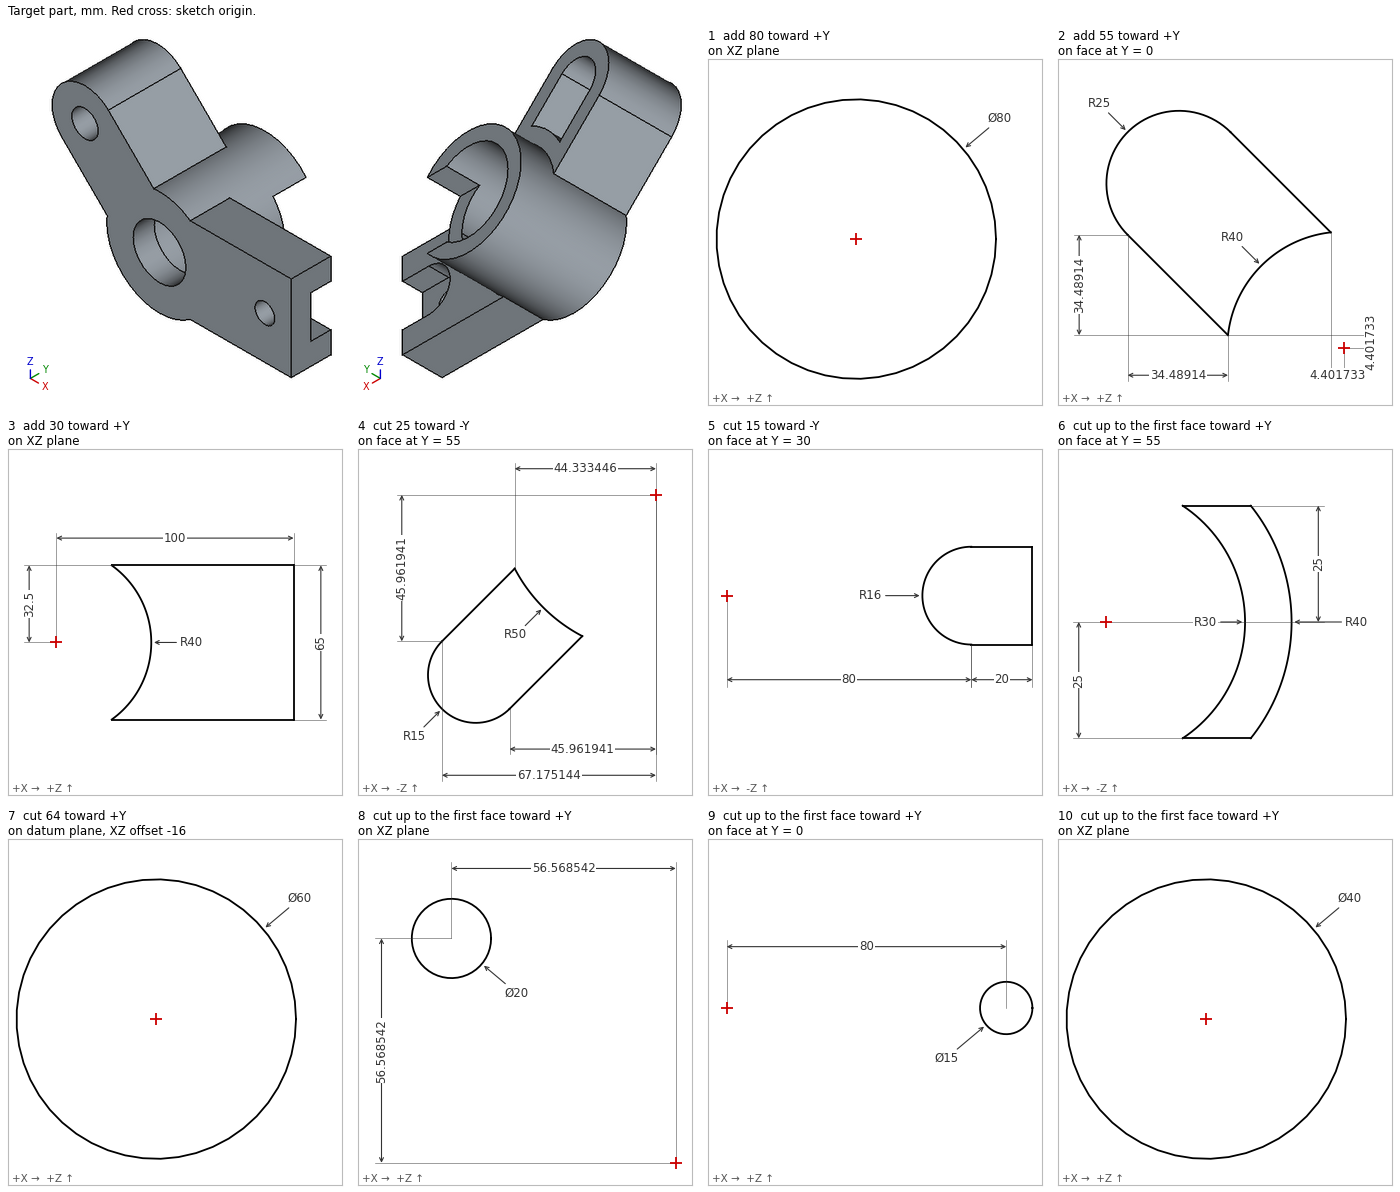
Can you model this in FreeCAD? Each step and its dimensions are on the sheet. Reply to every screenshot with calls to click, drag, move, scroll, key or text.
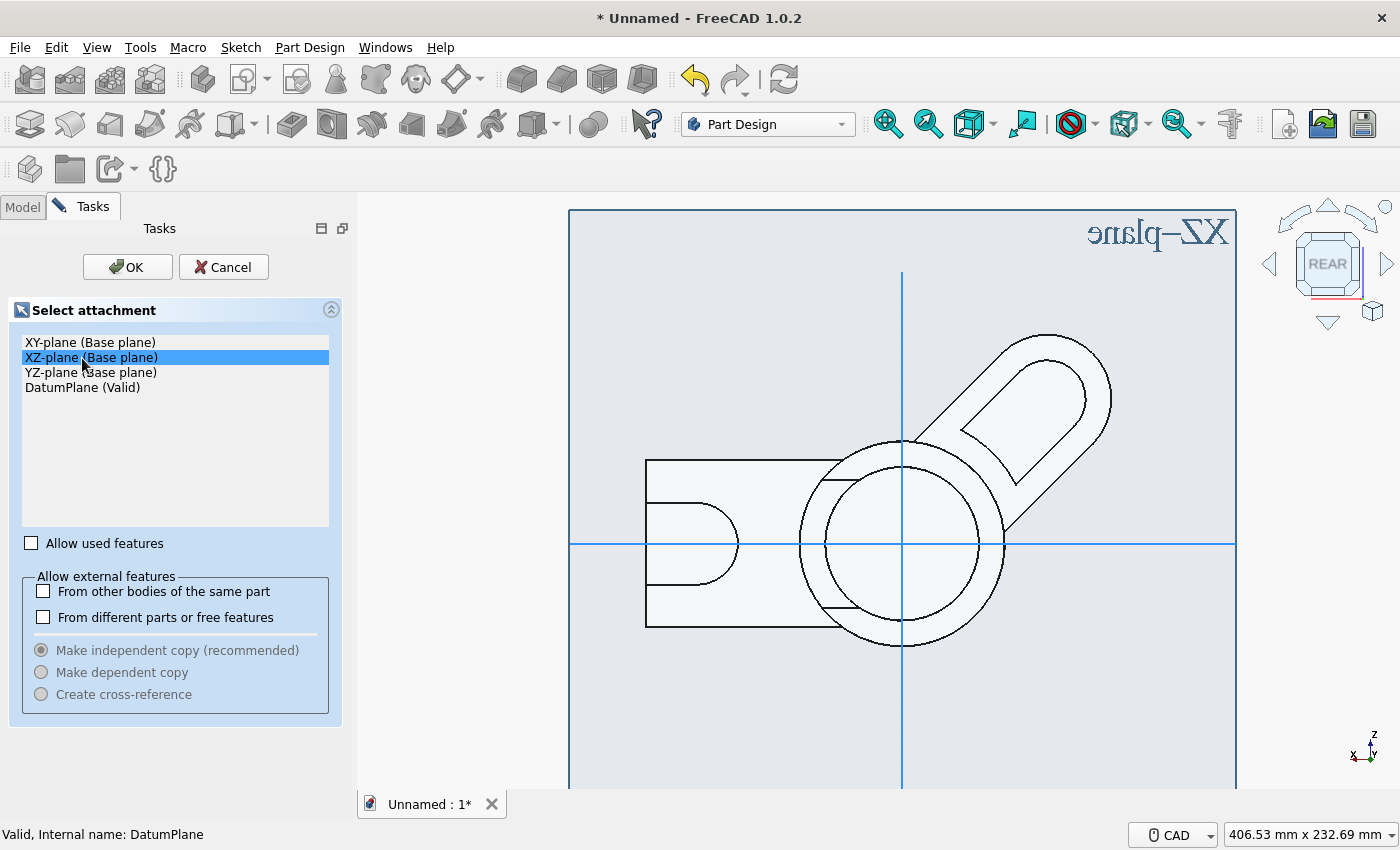
click(128, 267)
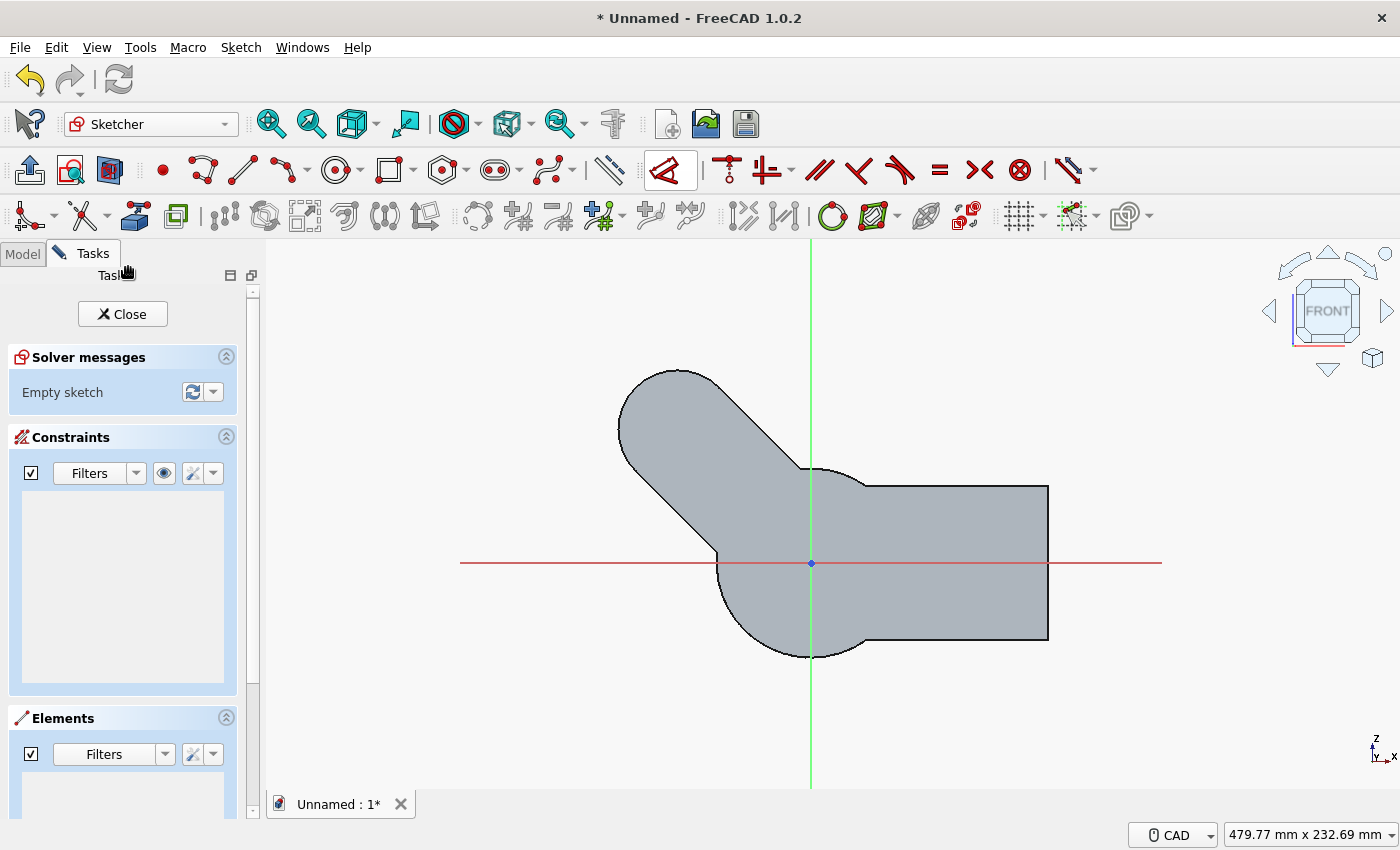
scroll(664, 416, up, 10)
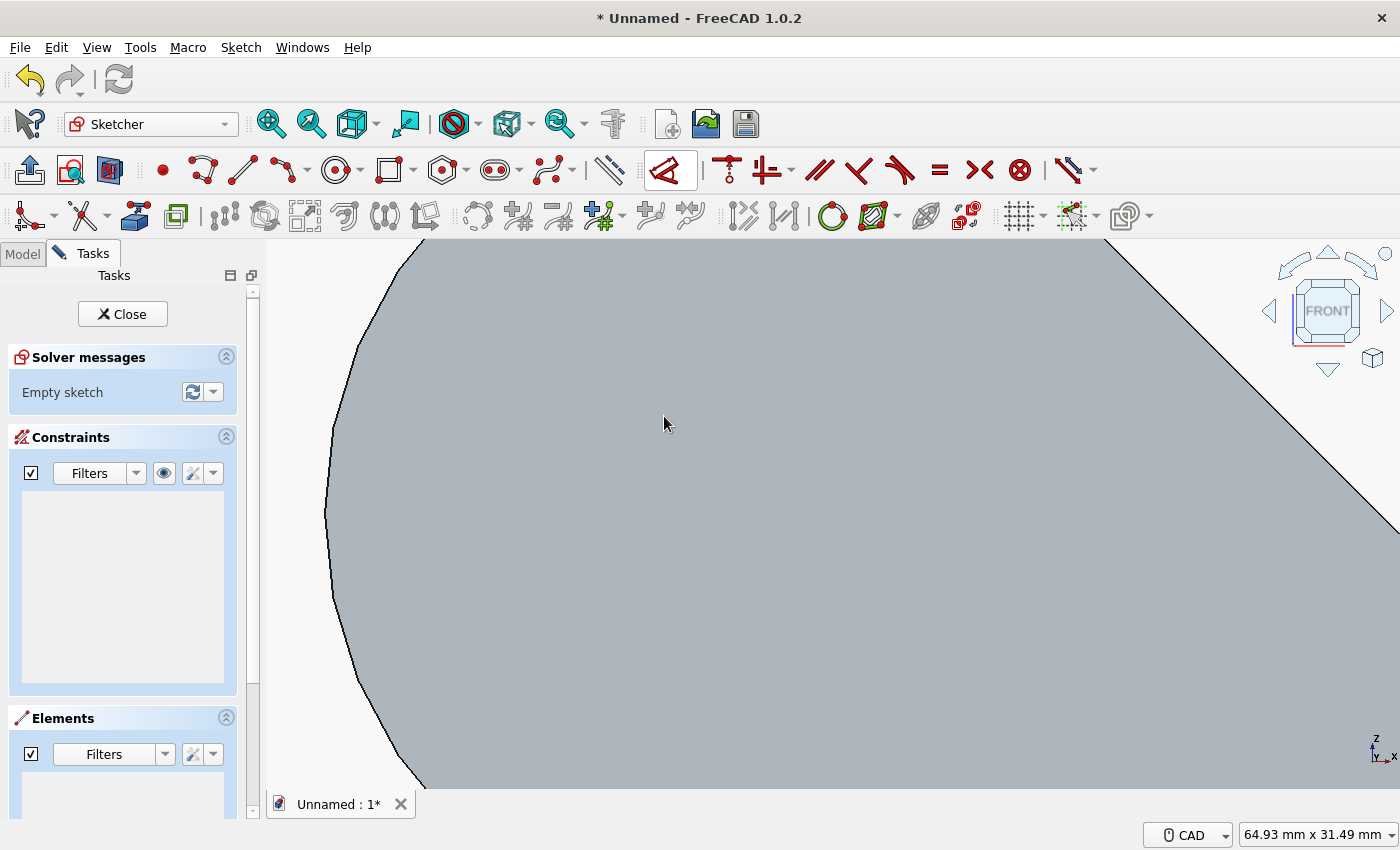
click(336, 170)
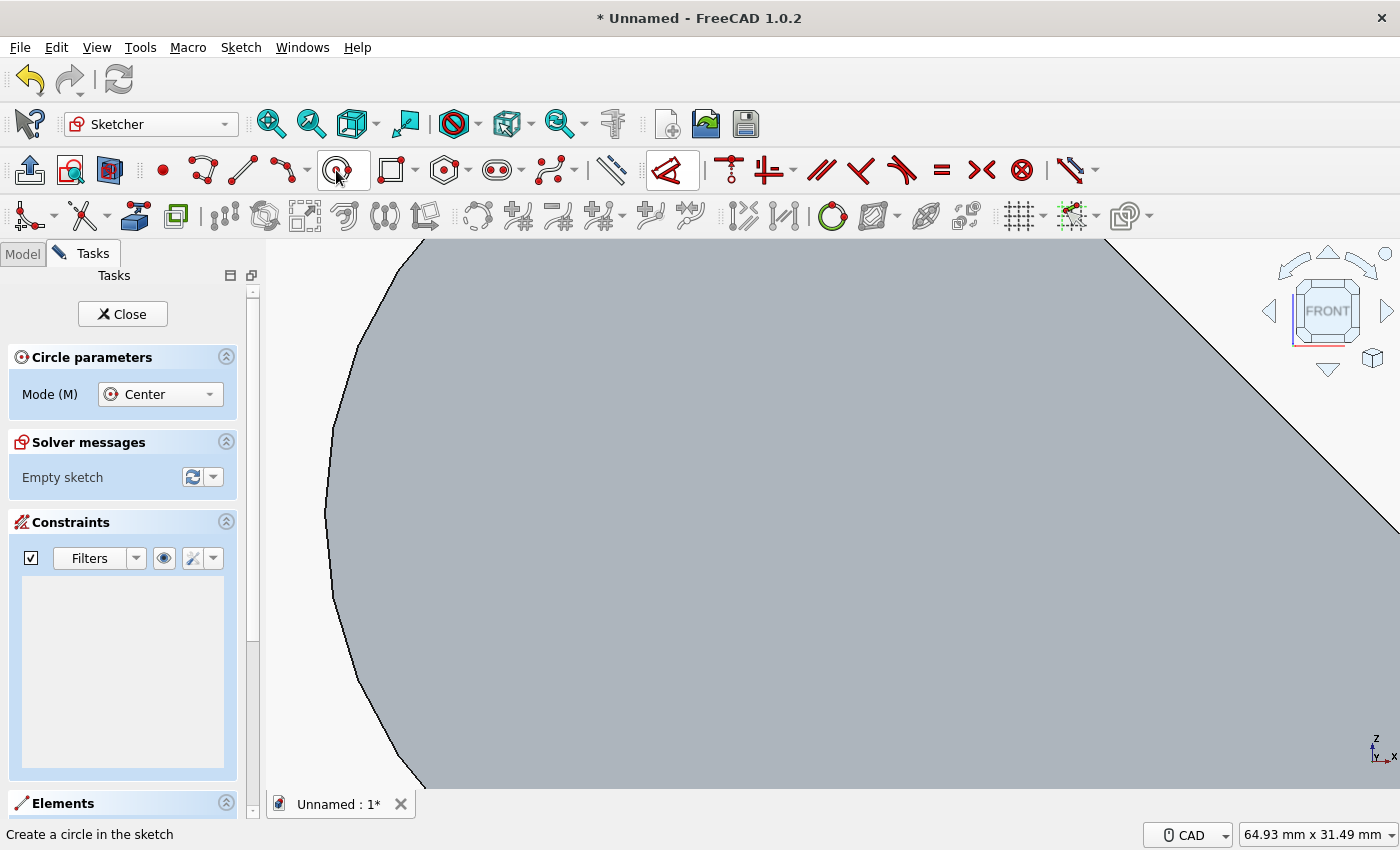
click(762, 513)
click(885, 390)
key(Escape)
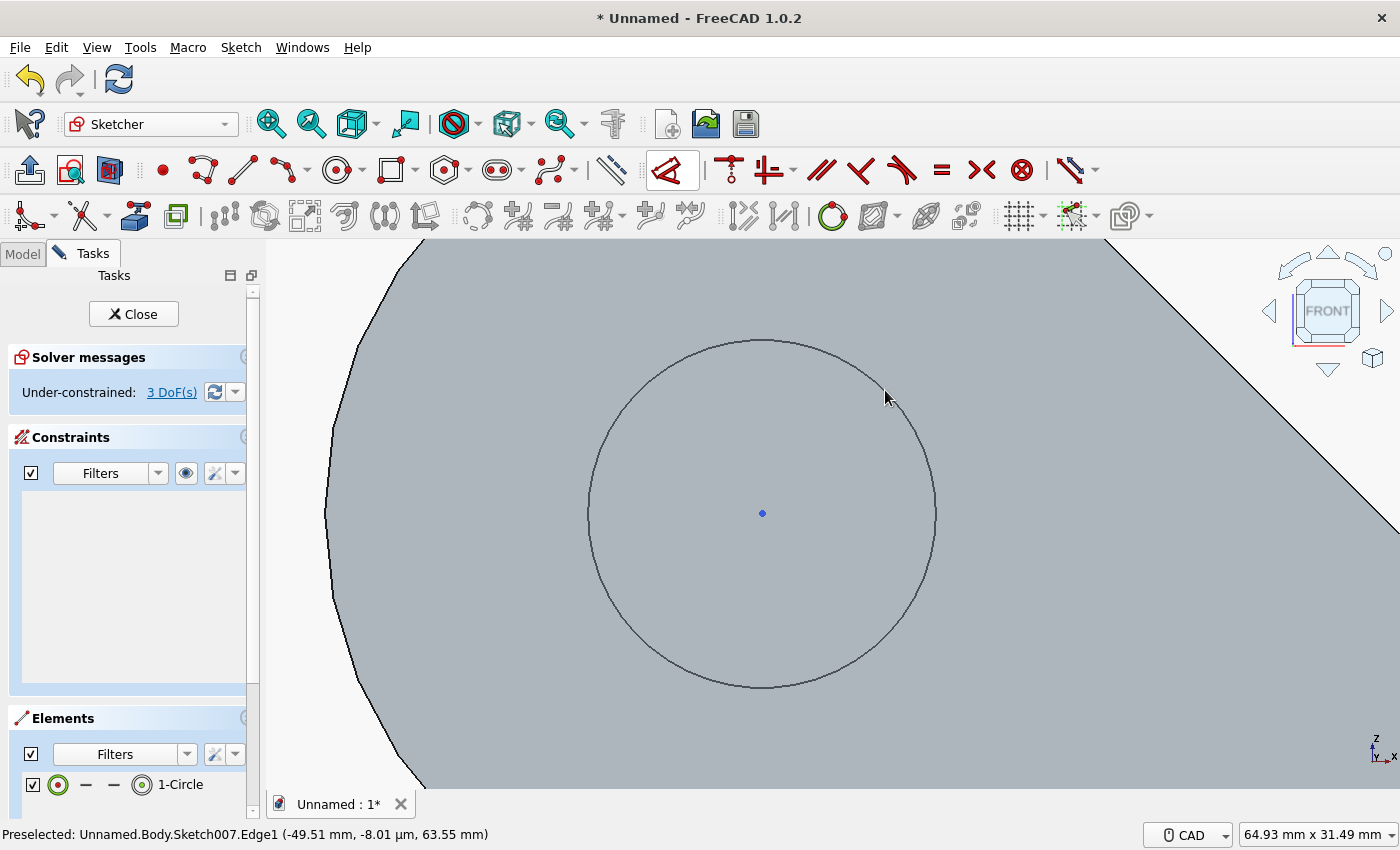
click(885, 391)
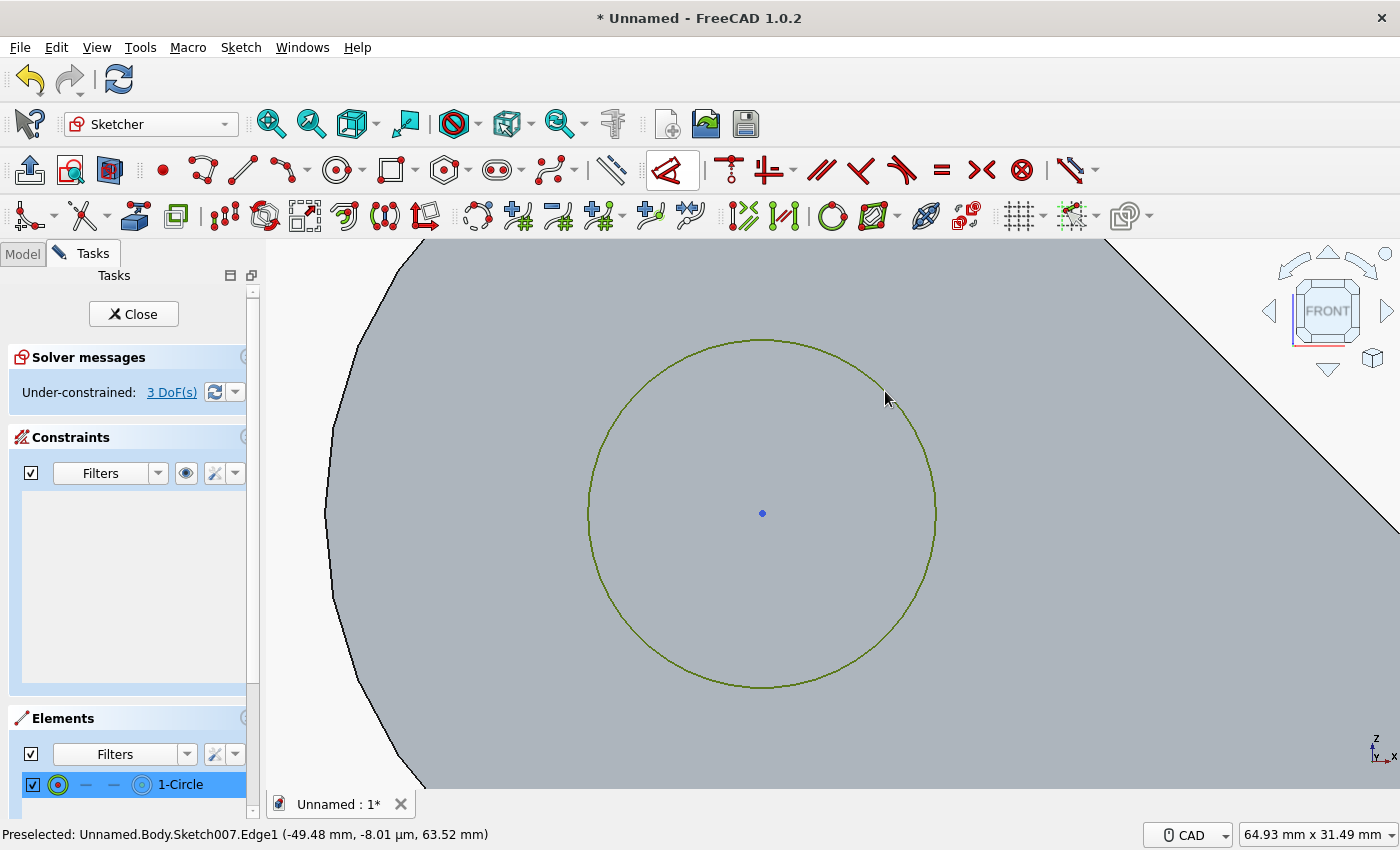
click(694, 170)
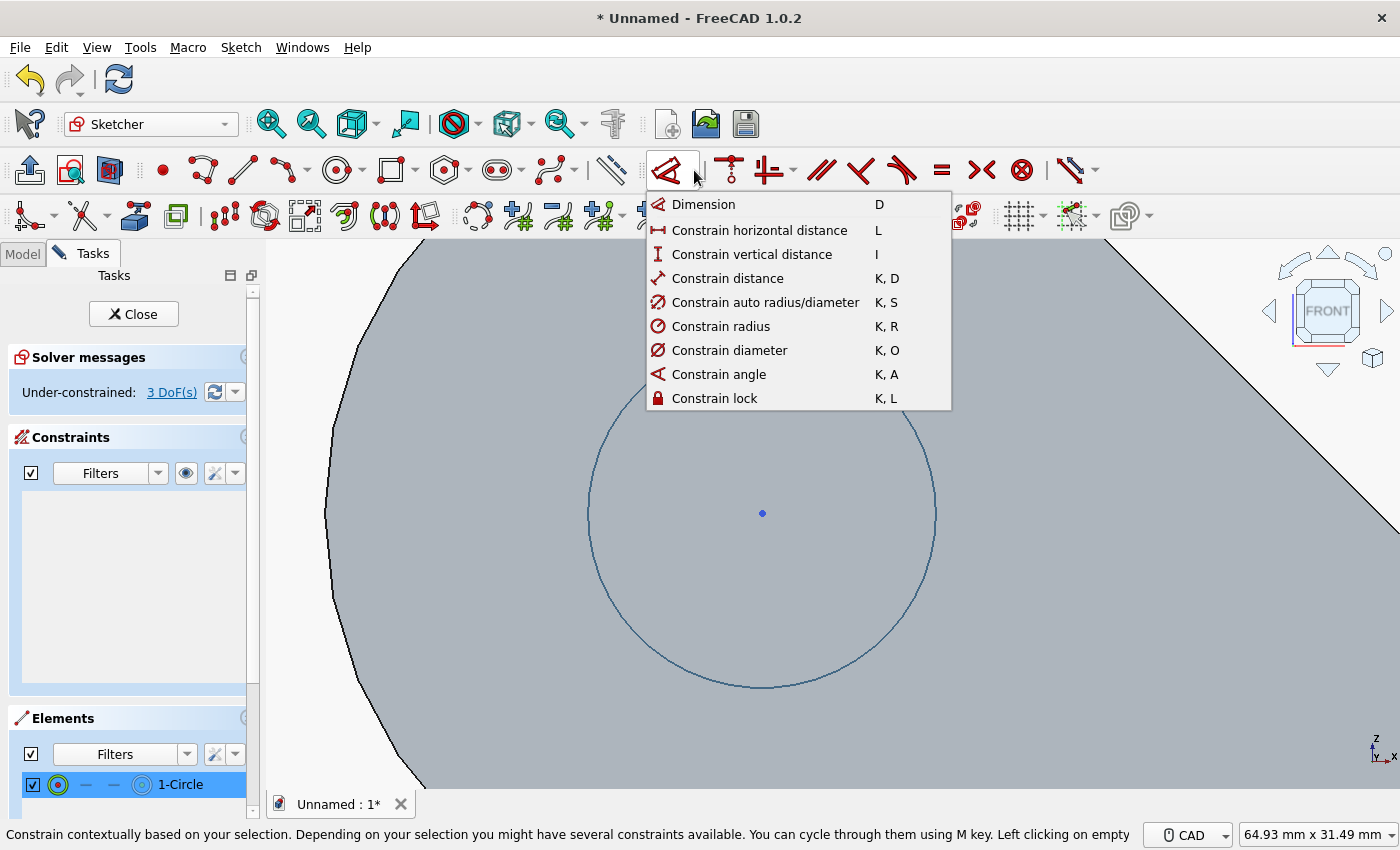
click(799, 350)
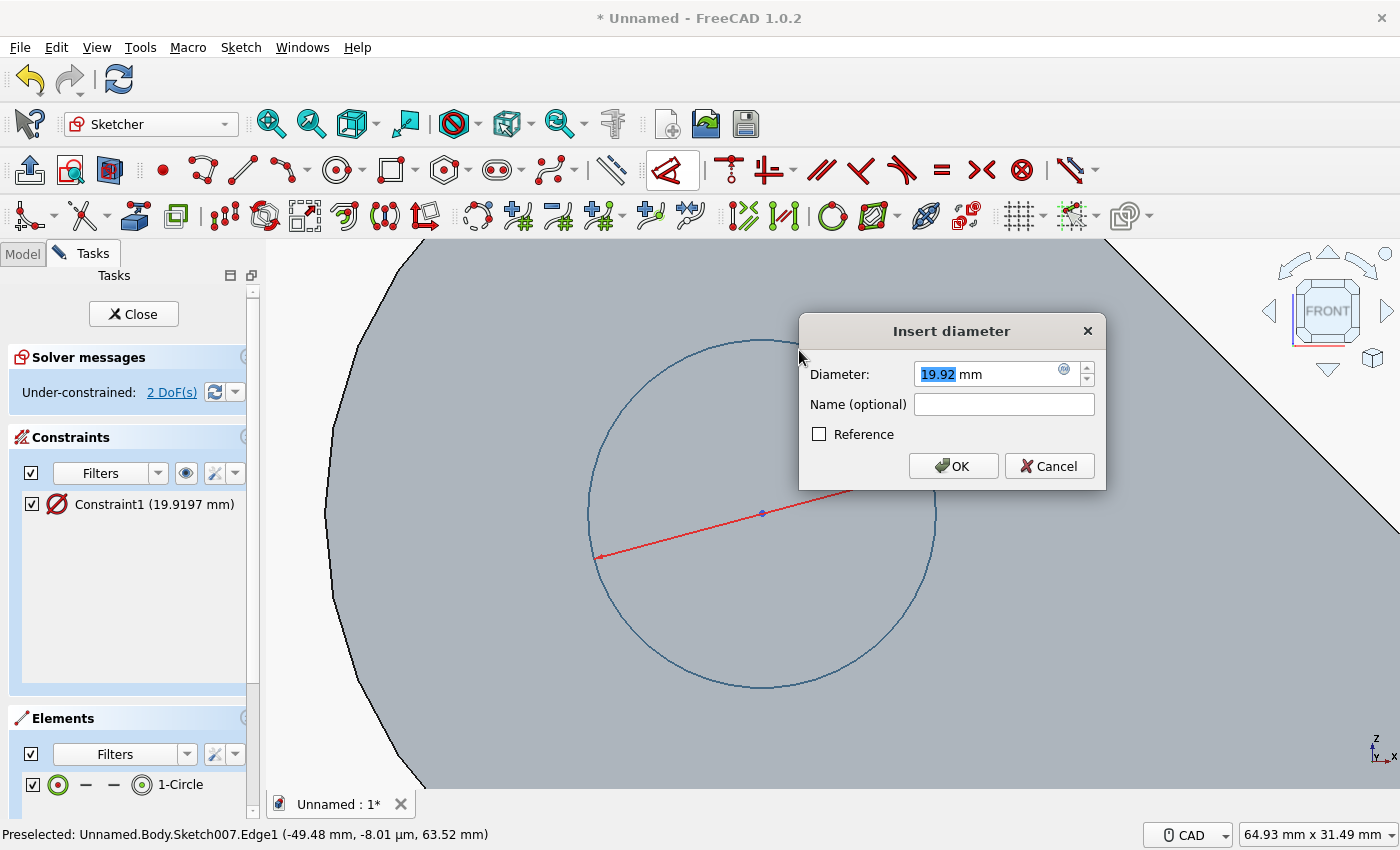
text(20)
key(Return)